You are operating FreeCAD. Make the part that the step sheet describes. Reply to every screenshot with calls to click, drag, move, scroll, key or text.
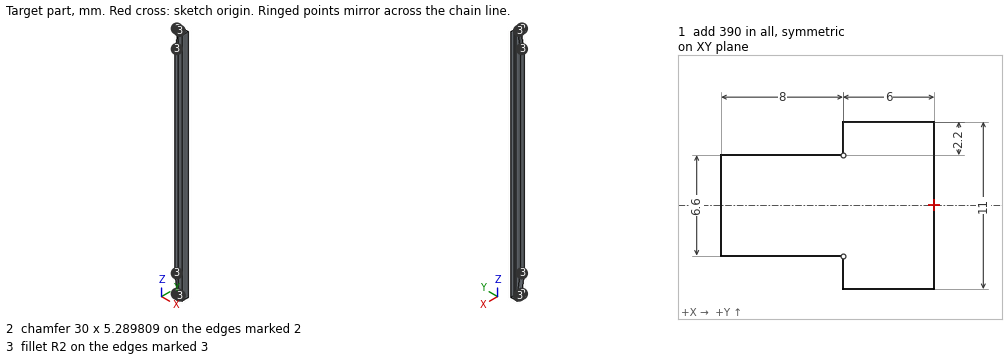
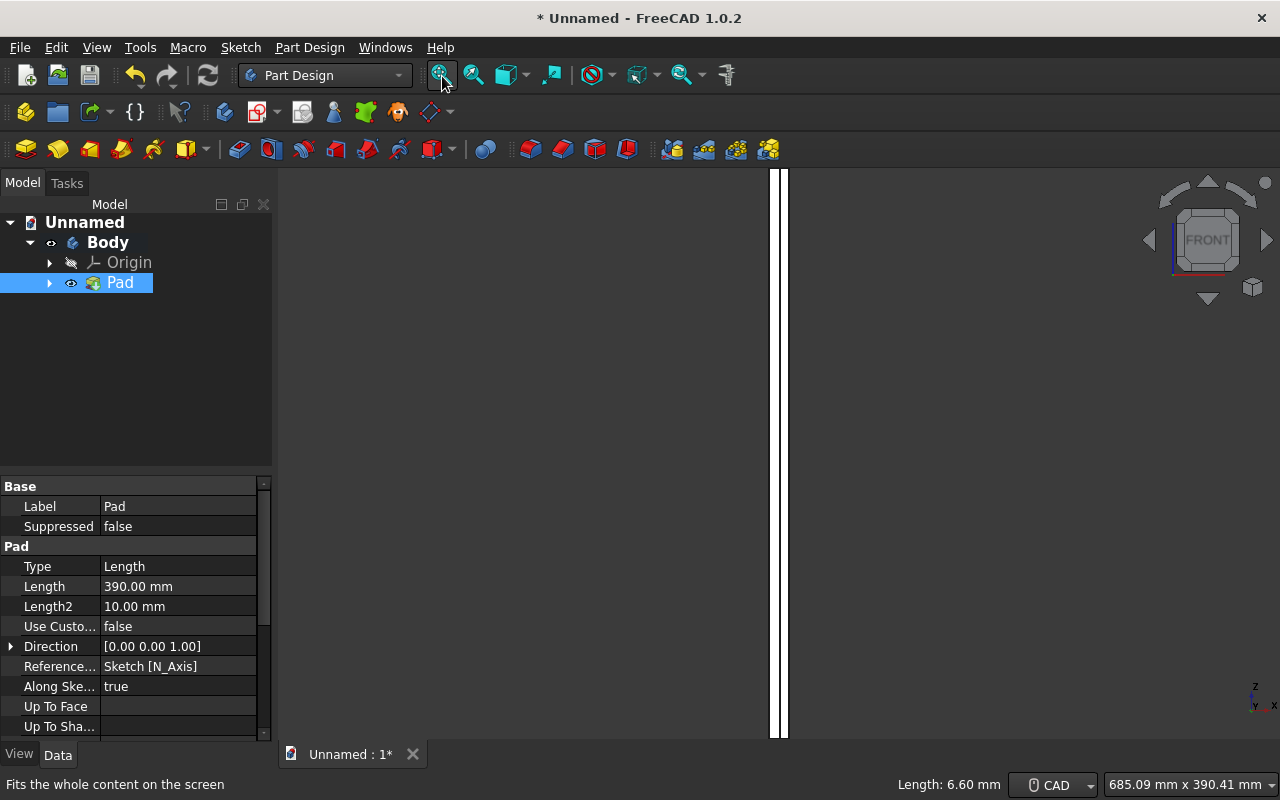
key(3)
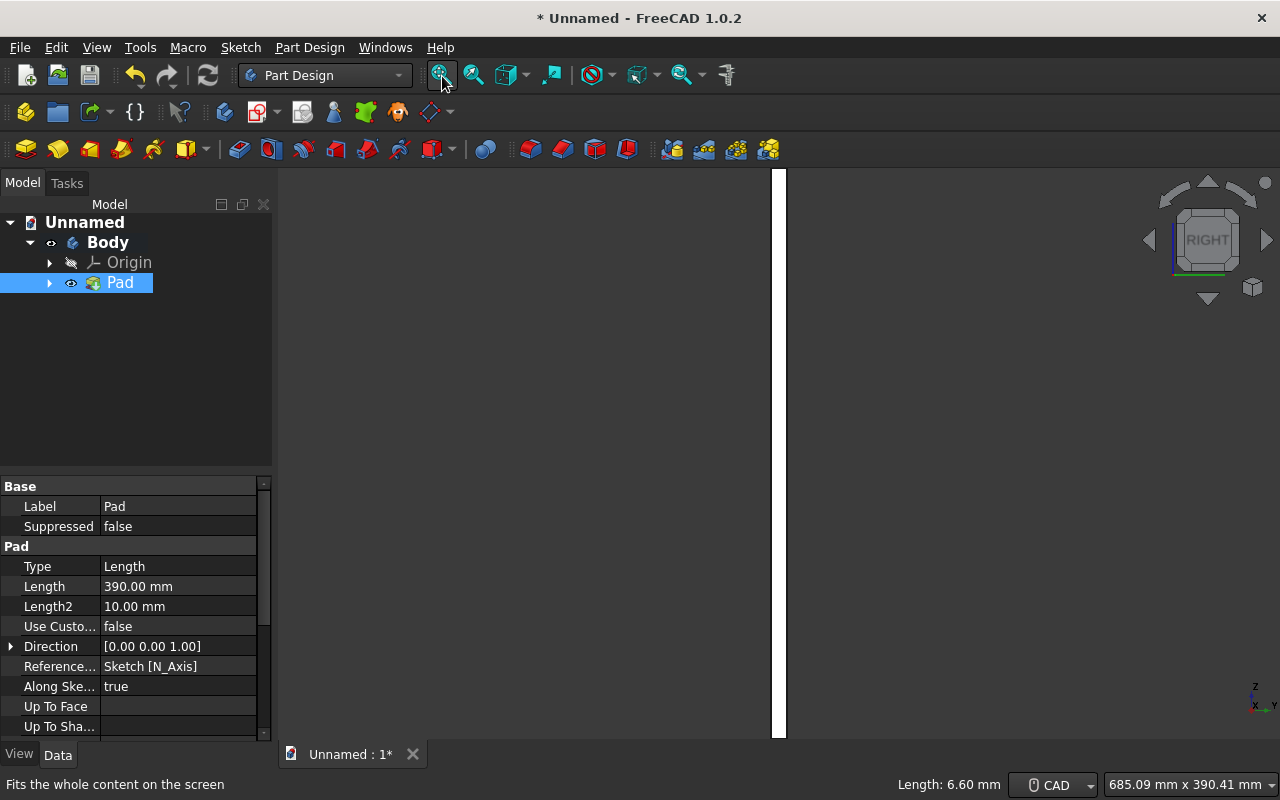
click(442, 76)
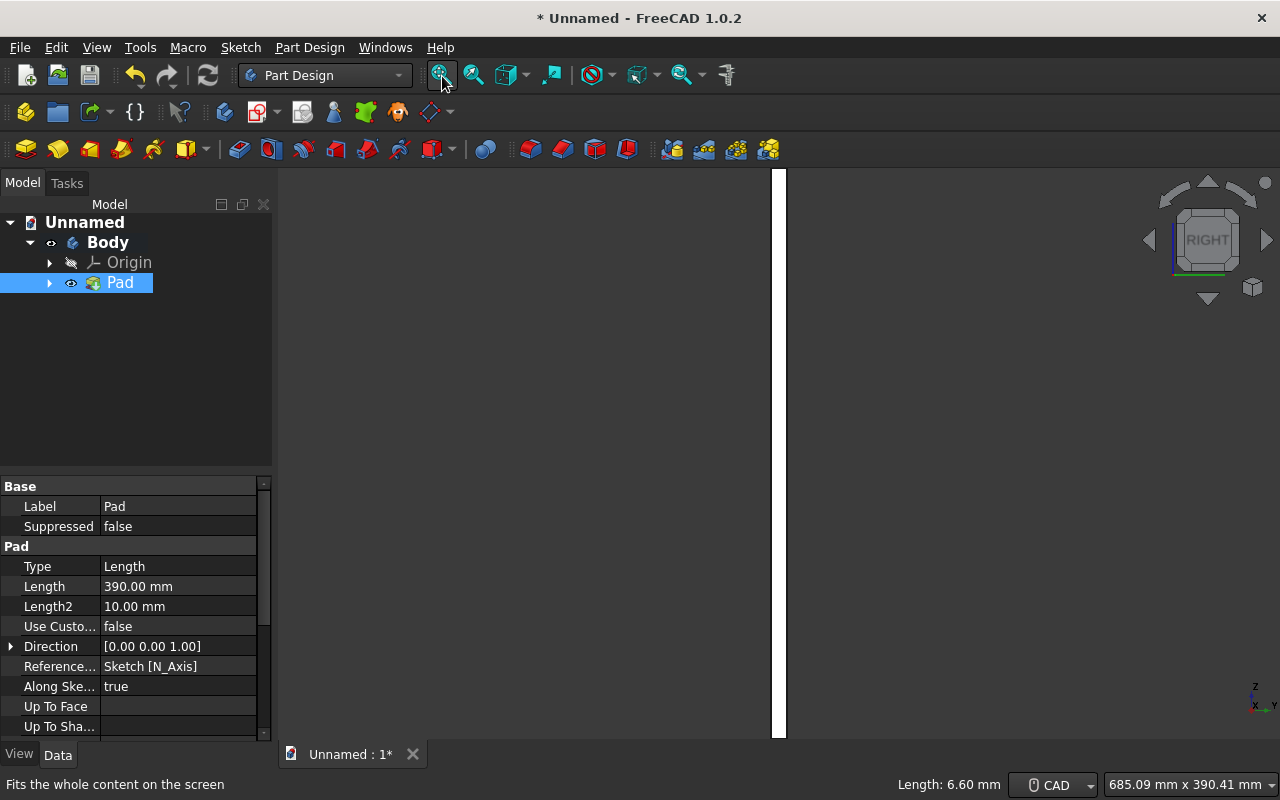
key(5)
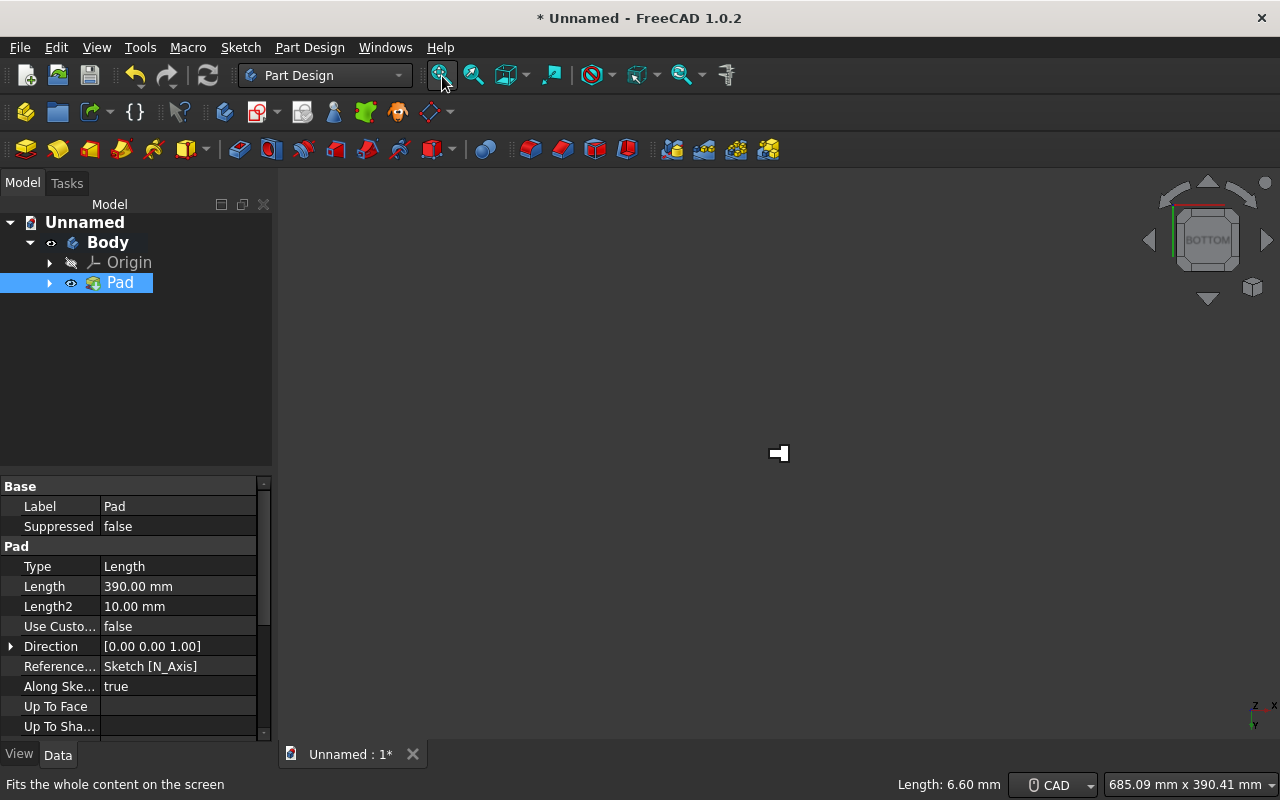
click(442, 76)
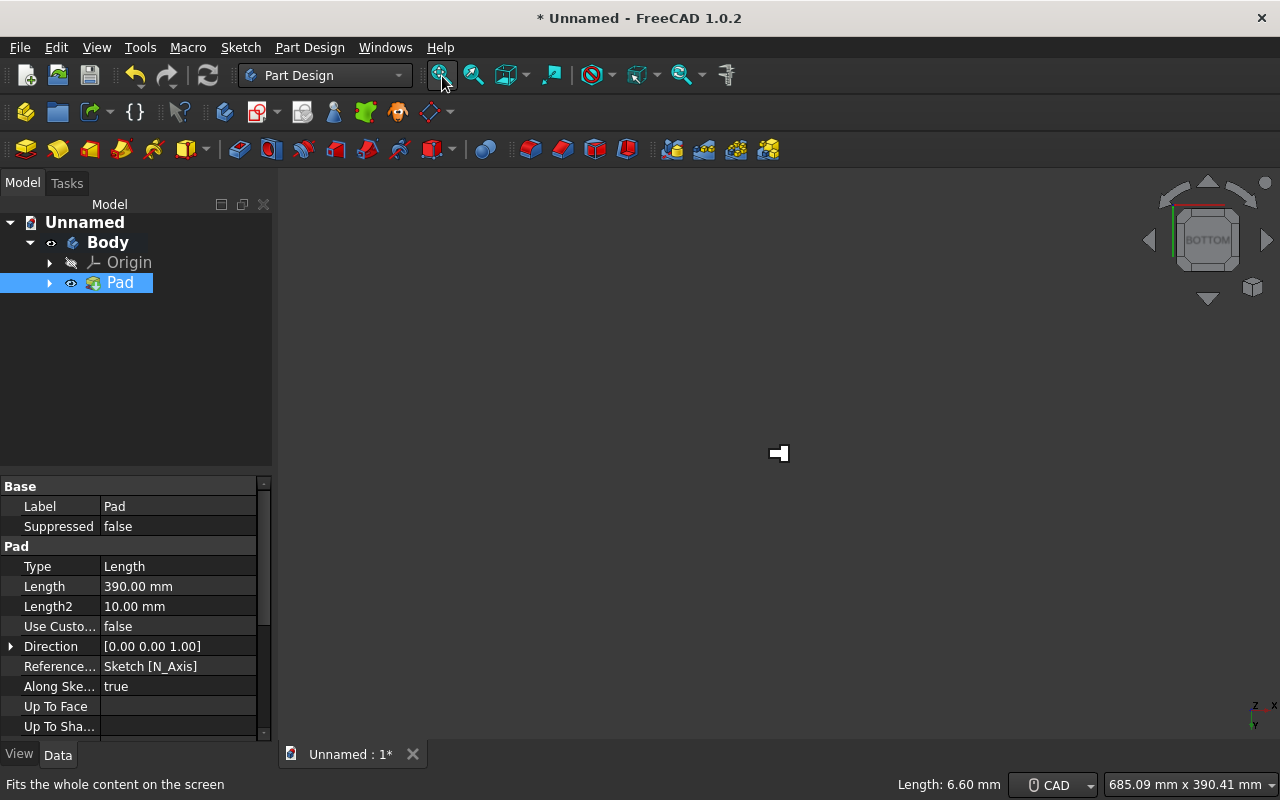
scroll(769, 452, up, 8)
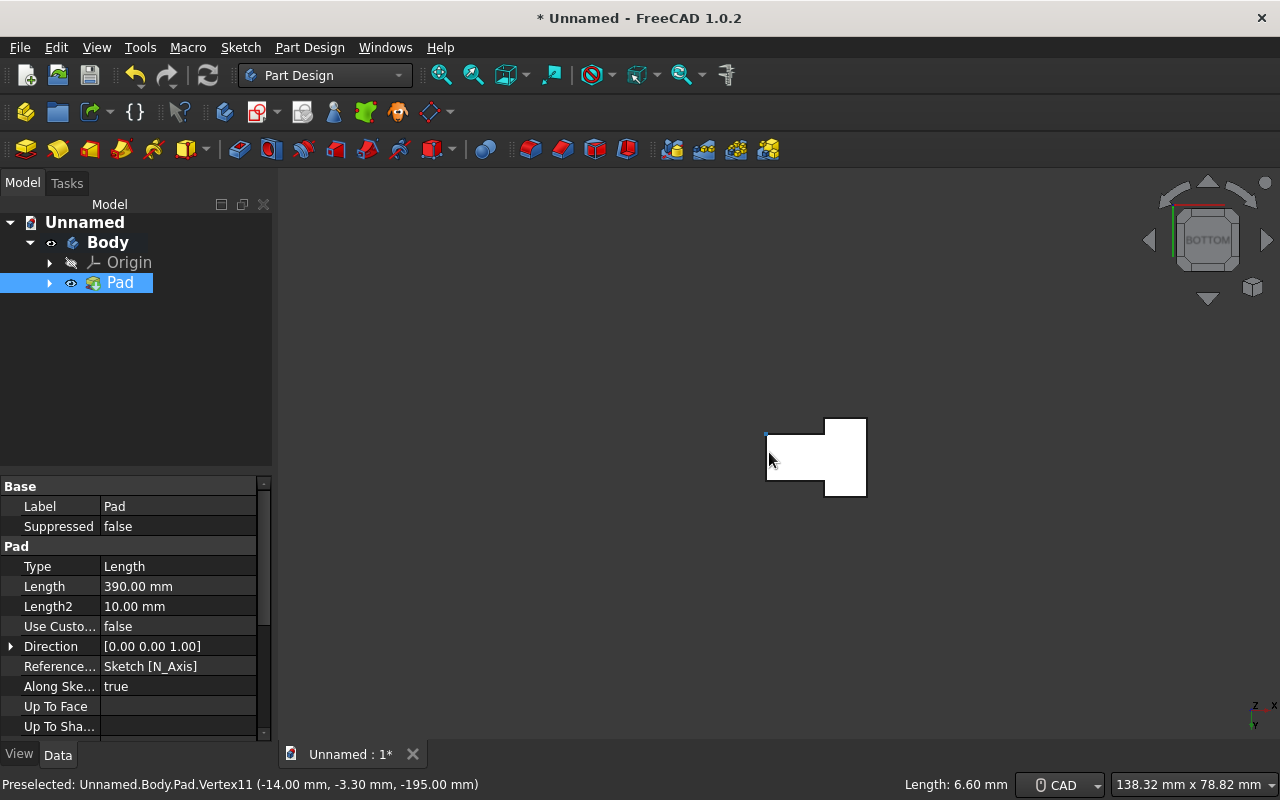
click(766, 456, ctrl)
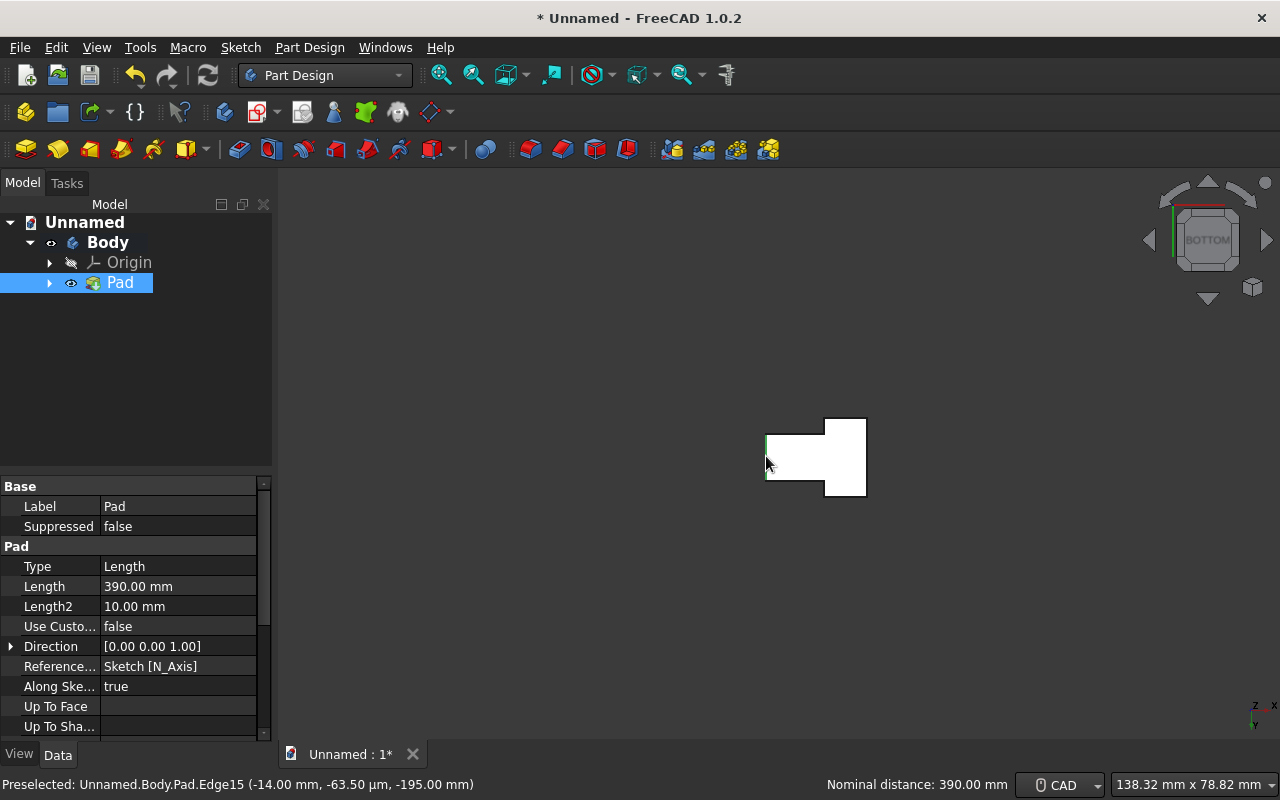
click(564, 150)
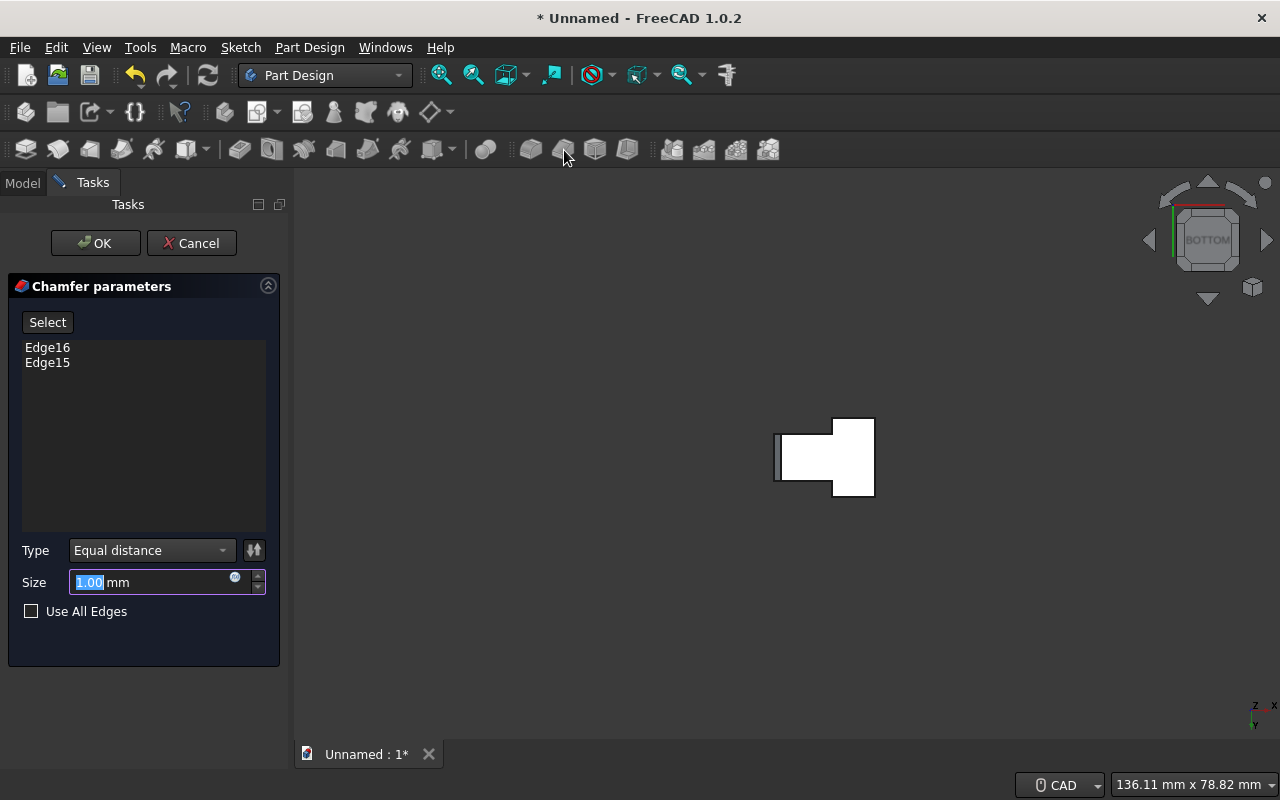
text(30)
key(Tab)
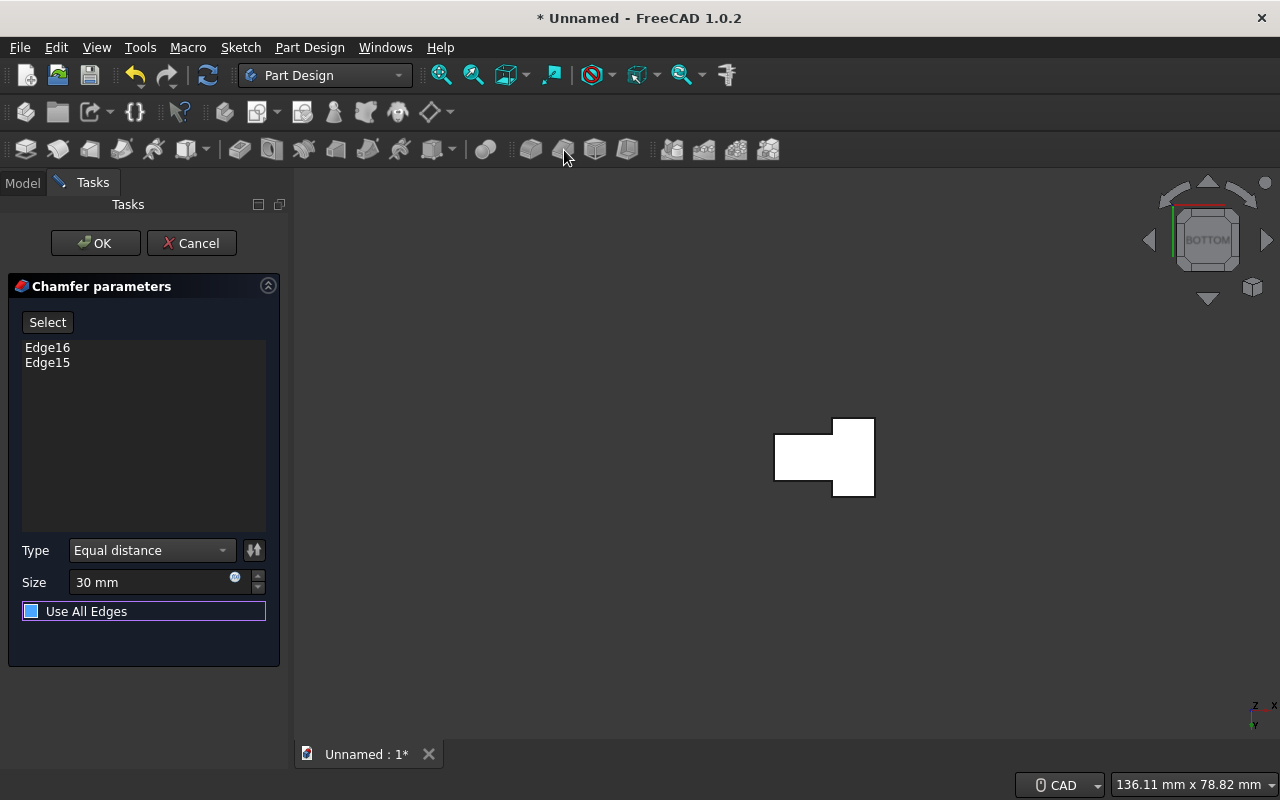
click(153, 550)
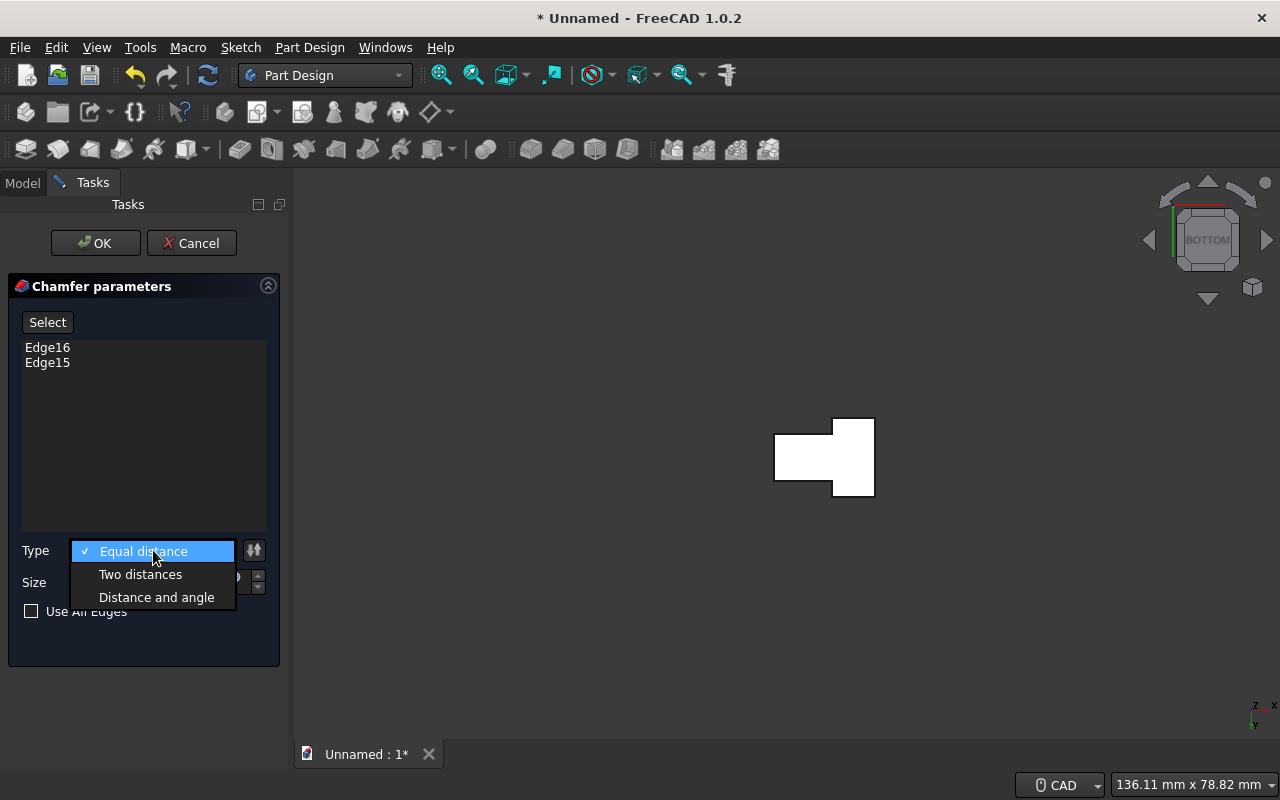
click(152, 574)